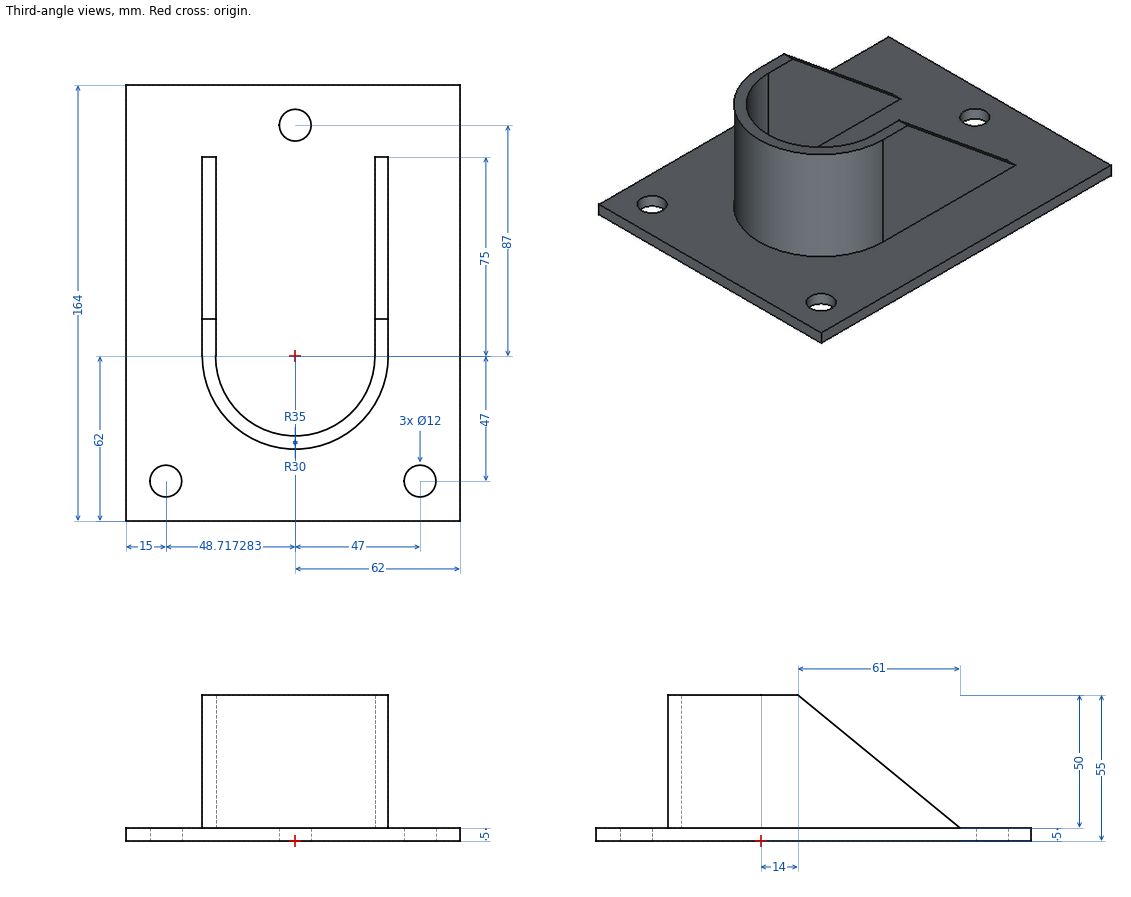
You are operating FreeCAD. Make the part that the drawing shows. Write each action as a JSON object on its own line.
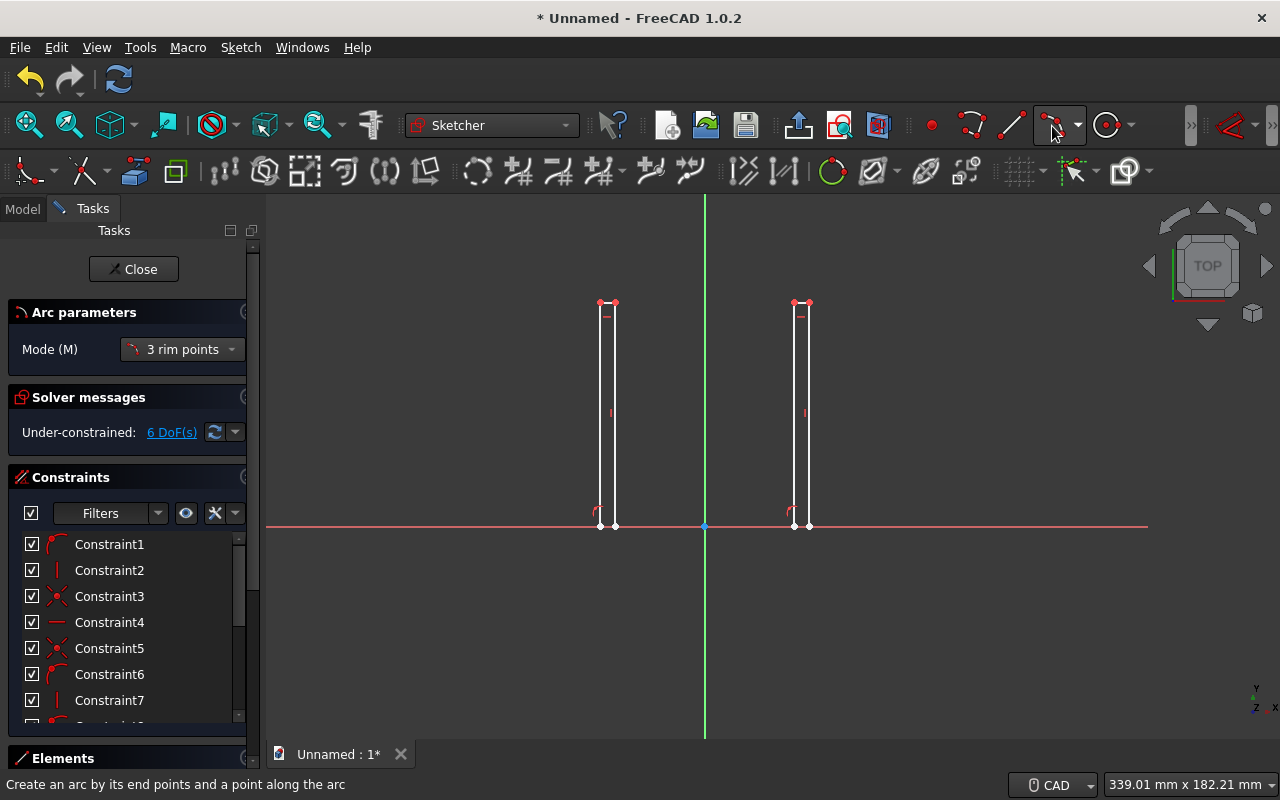
{"action": "left_click", "coordinate": [794, 527]}
{"action": "left_click", "coordinate": [615, 527]}
{"action": "left_click", "coordinate": [677, 612]}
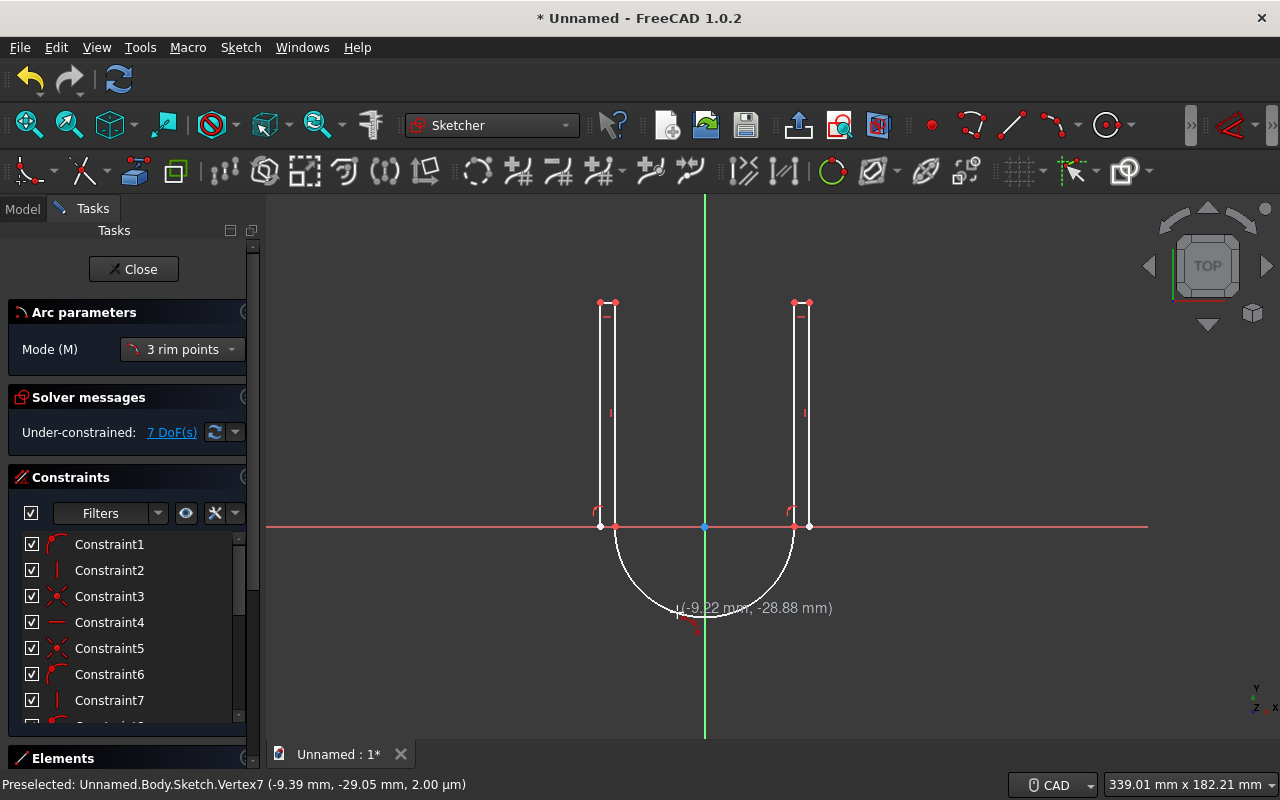
{"action": "left_click", "coordinate": [600, 527]}
{"action": "left_click", "coordinate": [809, 527]}
{"action": "left_click", "coordinate": [672, 626]}
{"action": "key", "text": "Escape"}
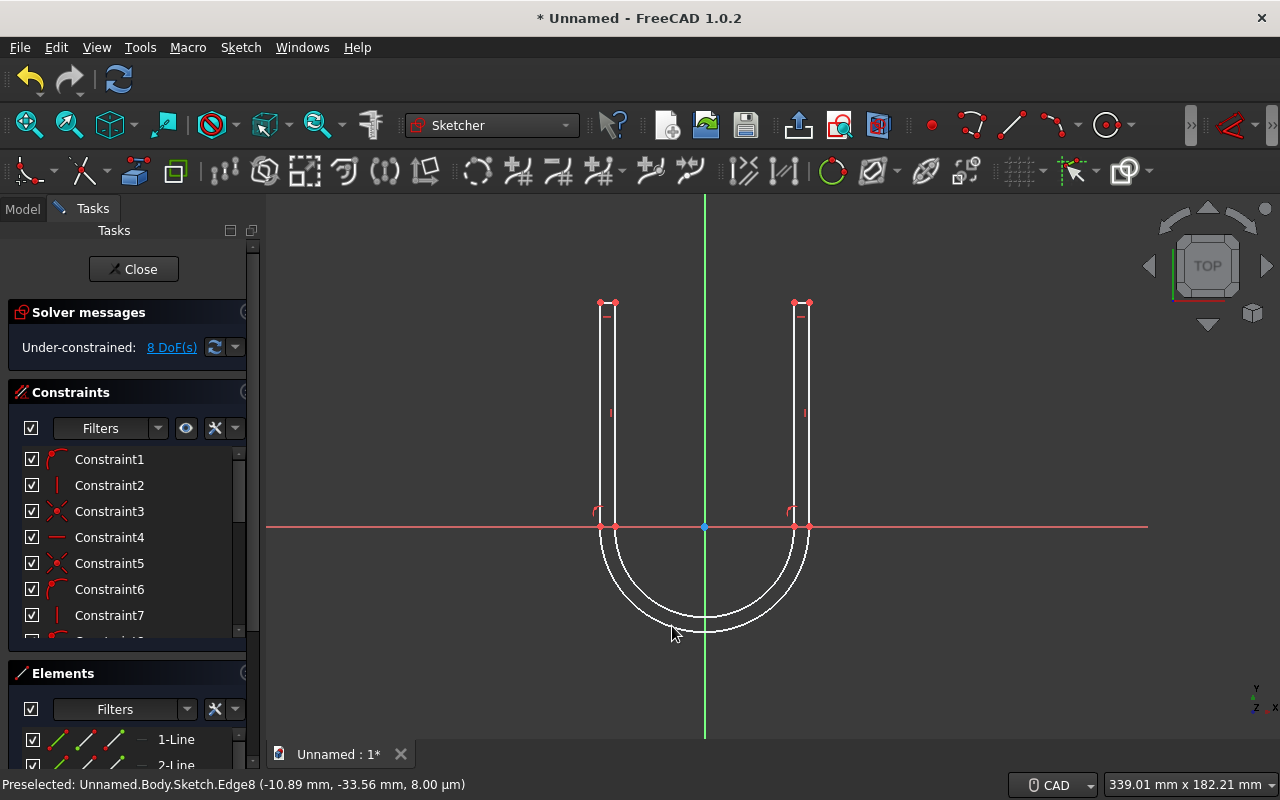
{"action": "left_click", "coordinate": [652, 600]}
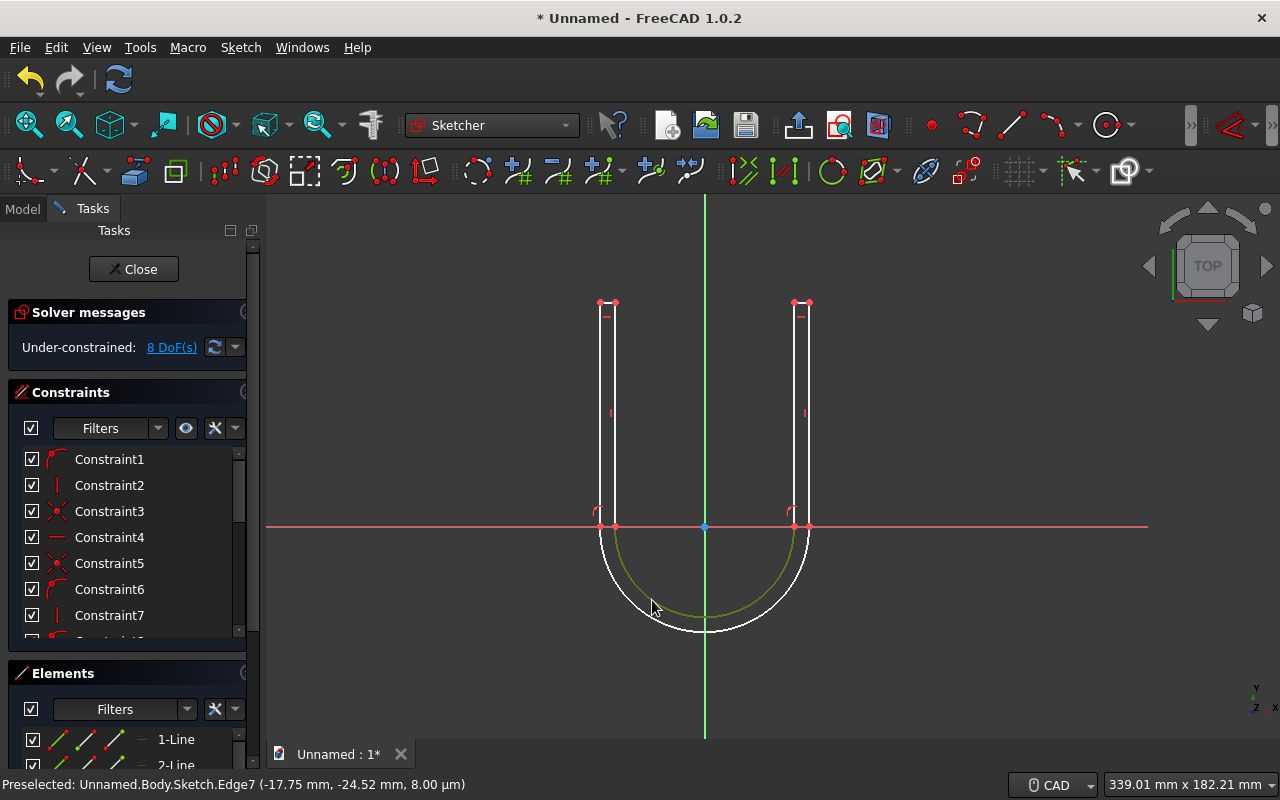
{"action": "left_click", "coordinate": [643, 612]}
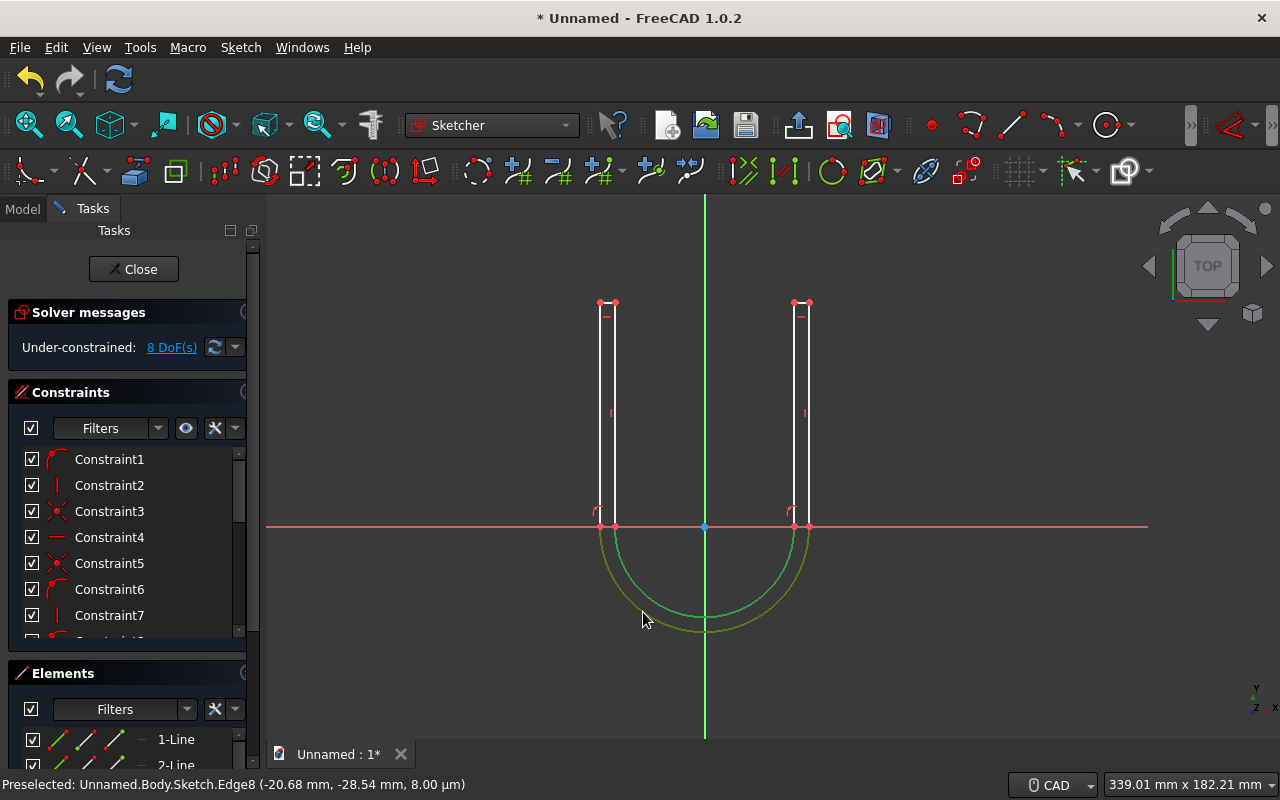
{"action": "key", "text": "c"}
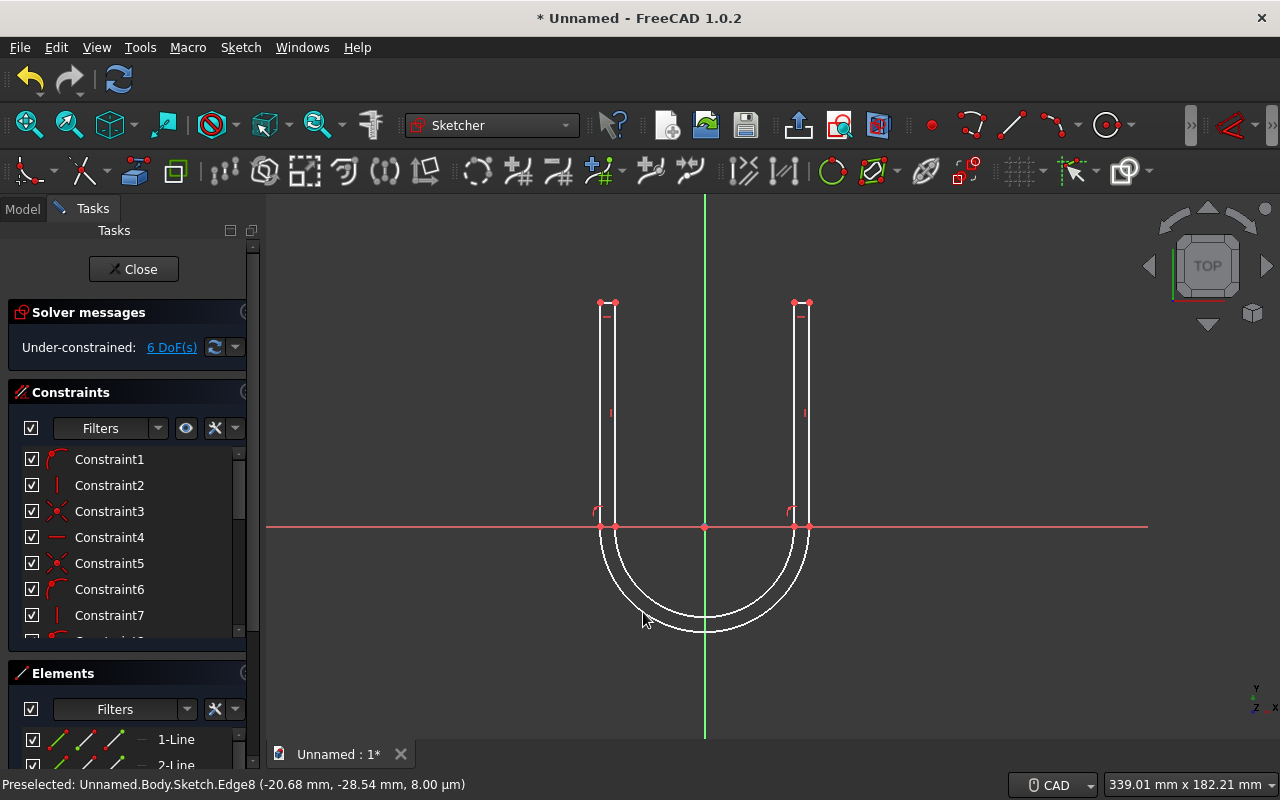
{"action": "left_click_drag", "start_coordinate": [695, 517], "coordinate": [715, 538]}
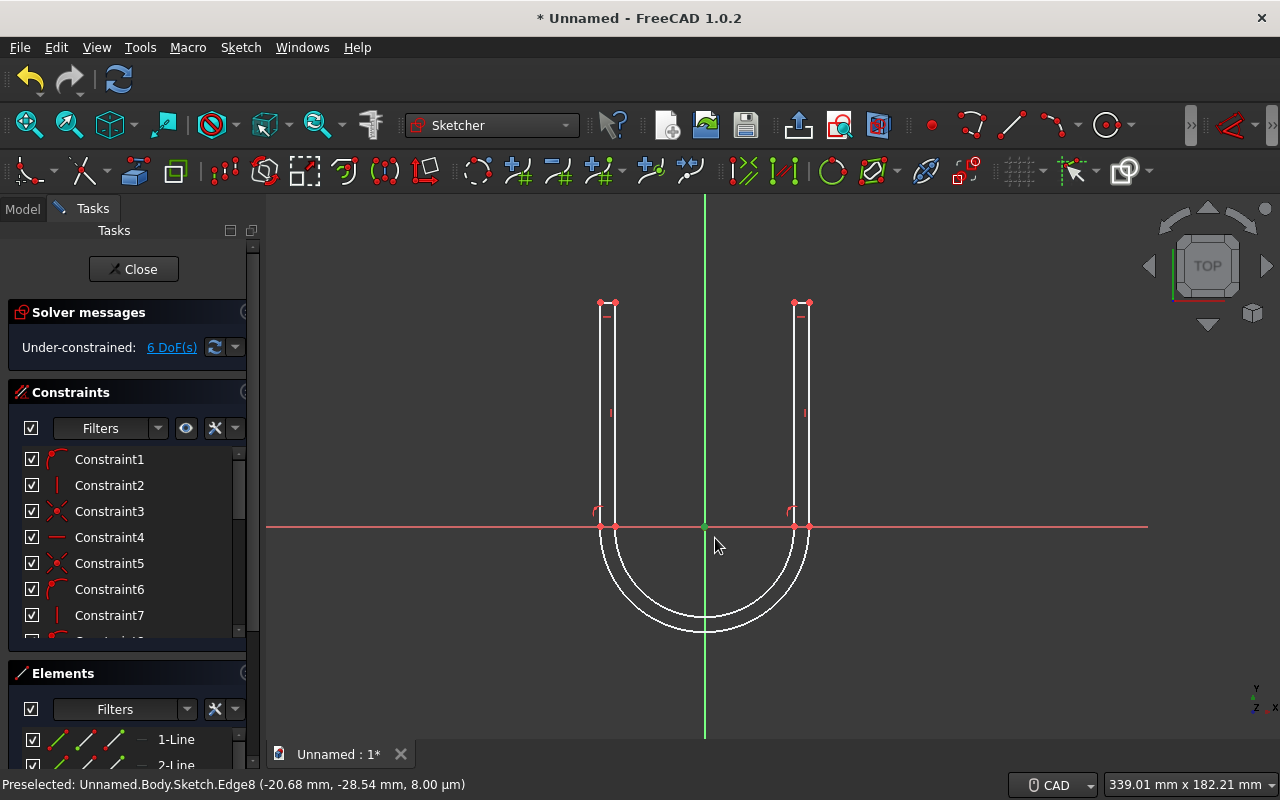
{"action": "key", "text": "c"}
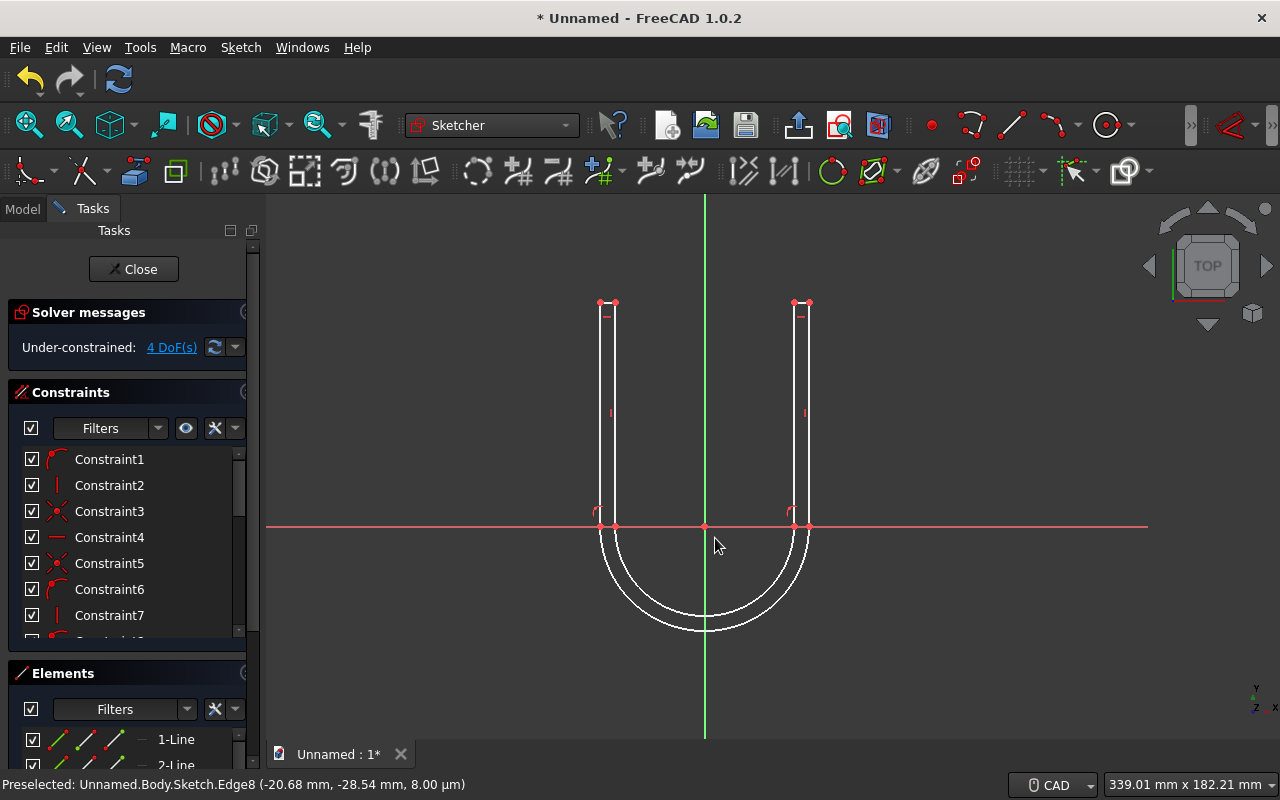
{"action": "left_click", "coordinate": [652, 599]}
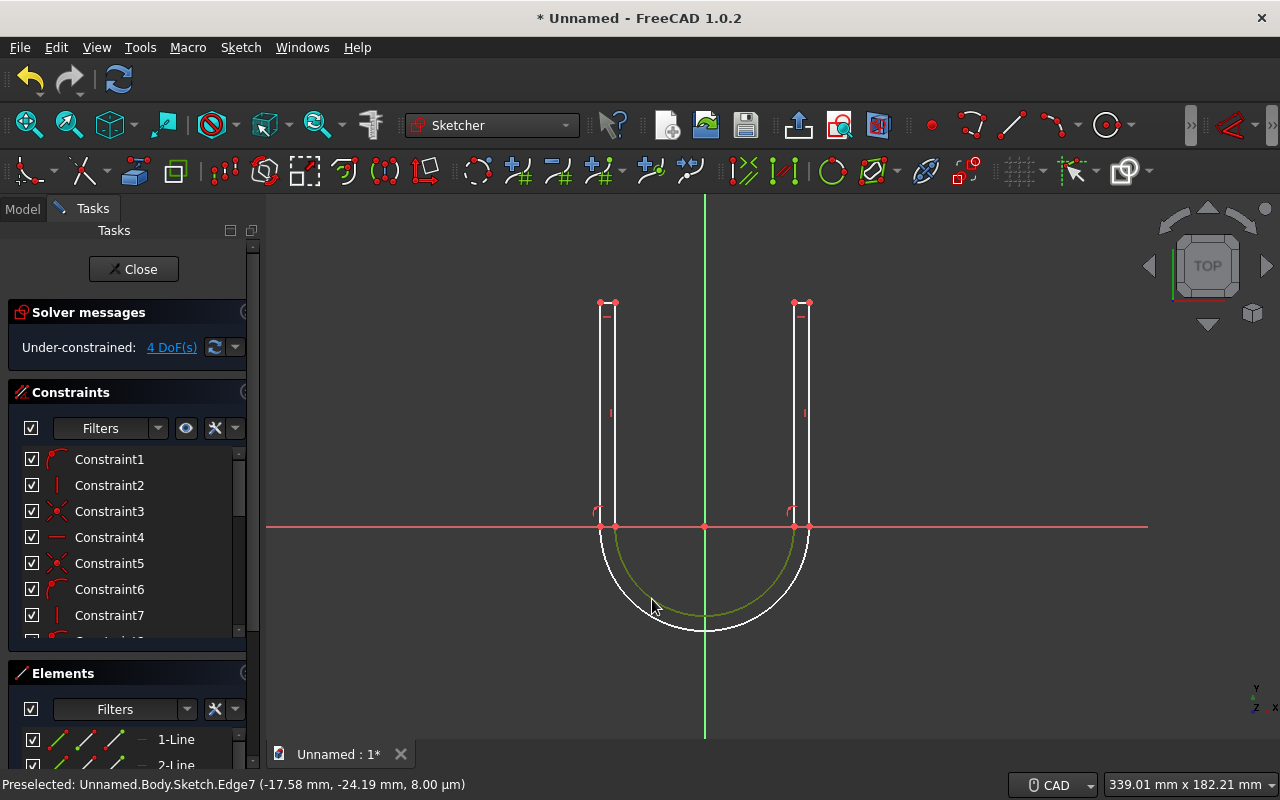
{"action": "left_click", "coordinate": [1258, 126]}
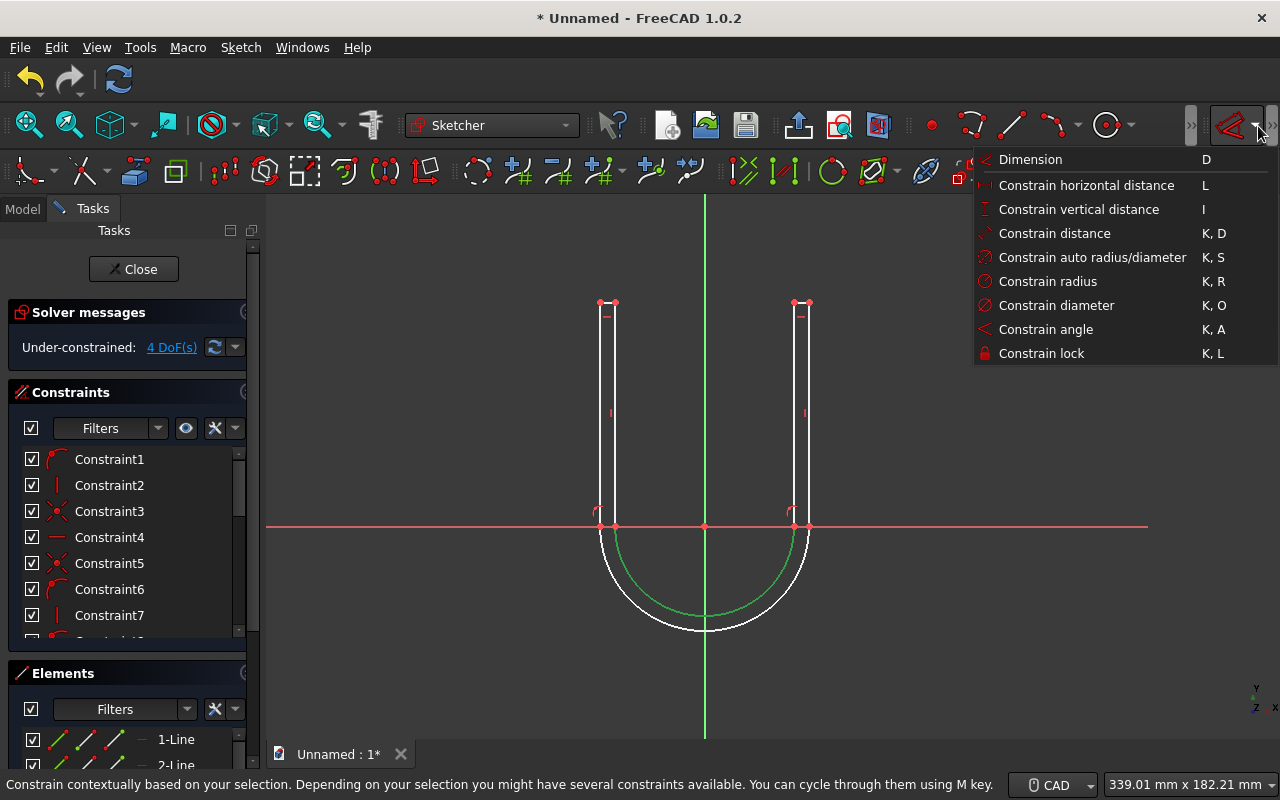
{"action": "left_click", "coordinate": [1126, 281]}